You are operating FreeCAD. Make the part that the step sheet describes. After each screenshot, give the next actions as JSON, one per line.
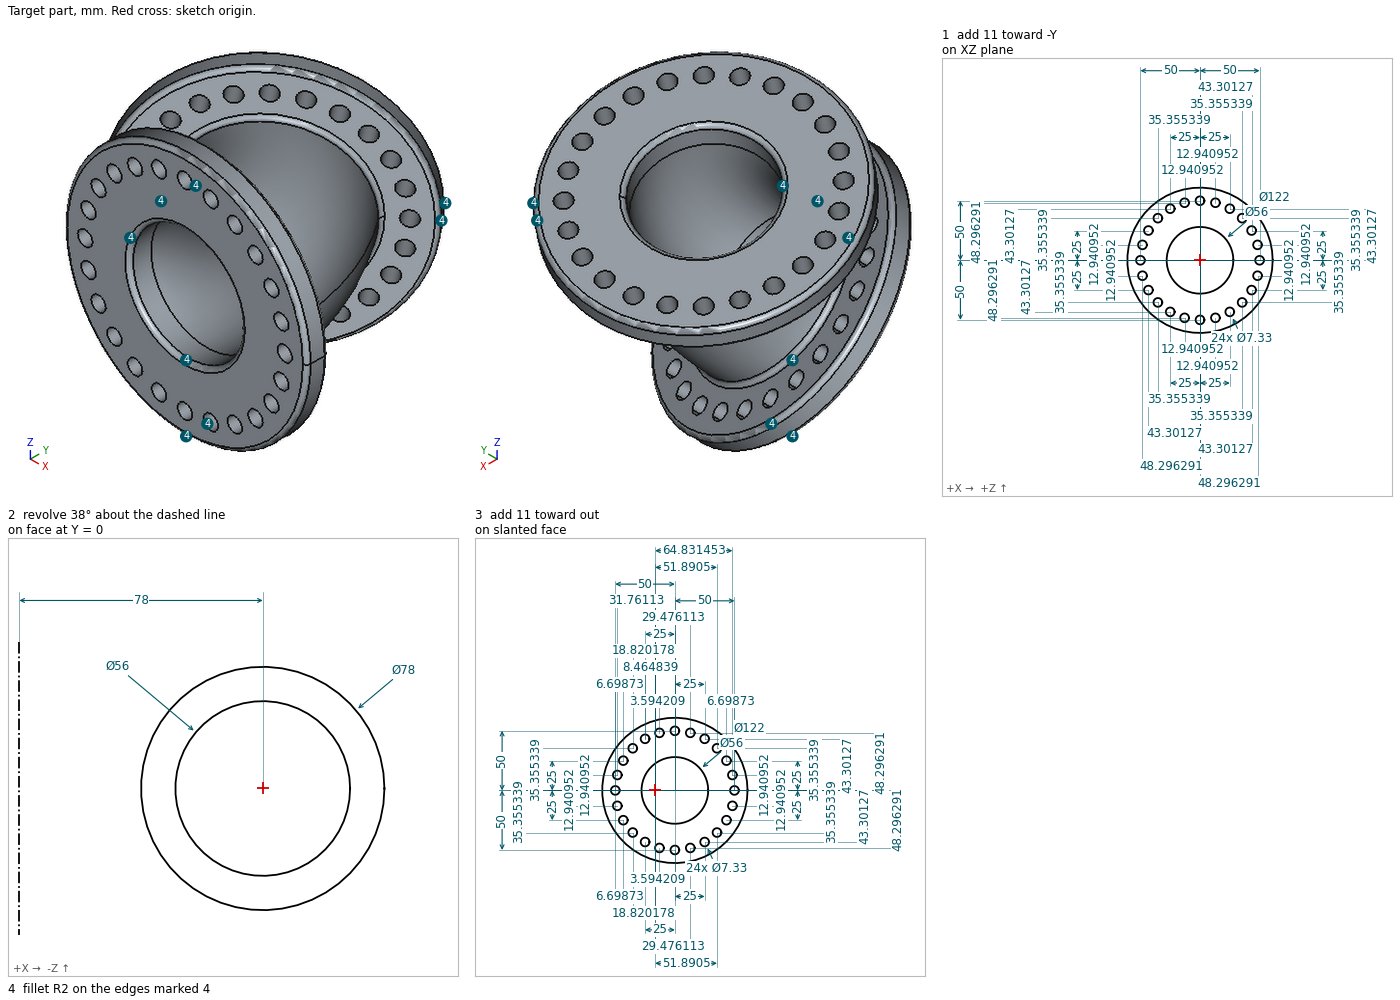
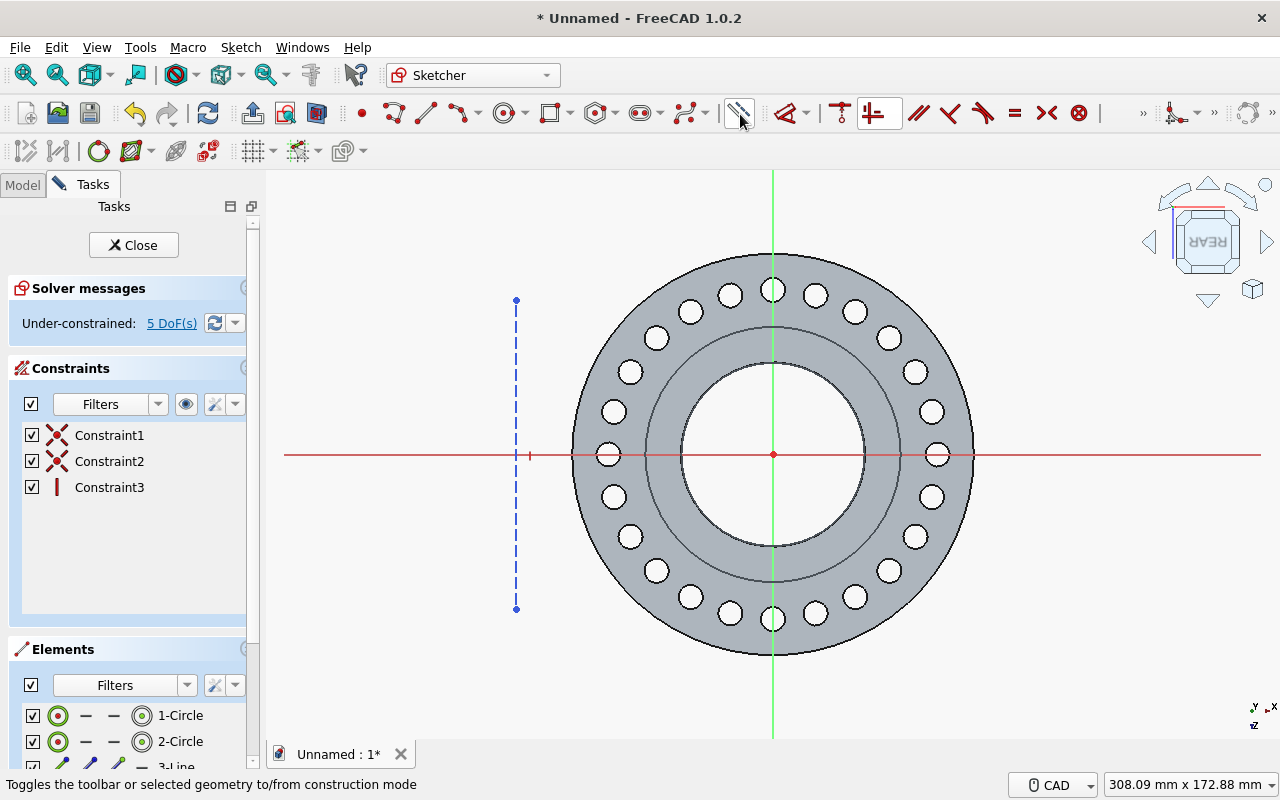
{"action": "left_click", "coordinate": [786, 114]}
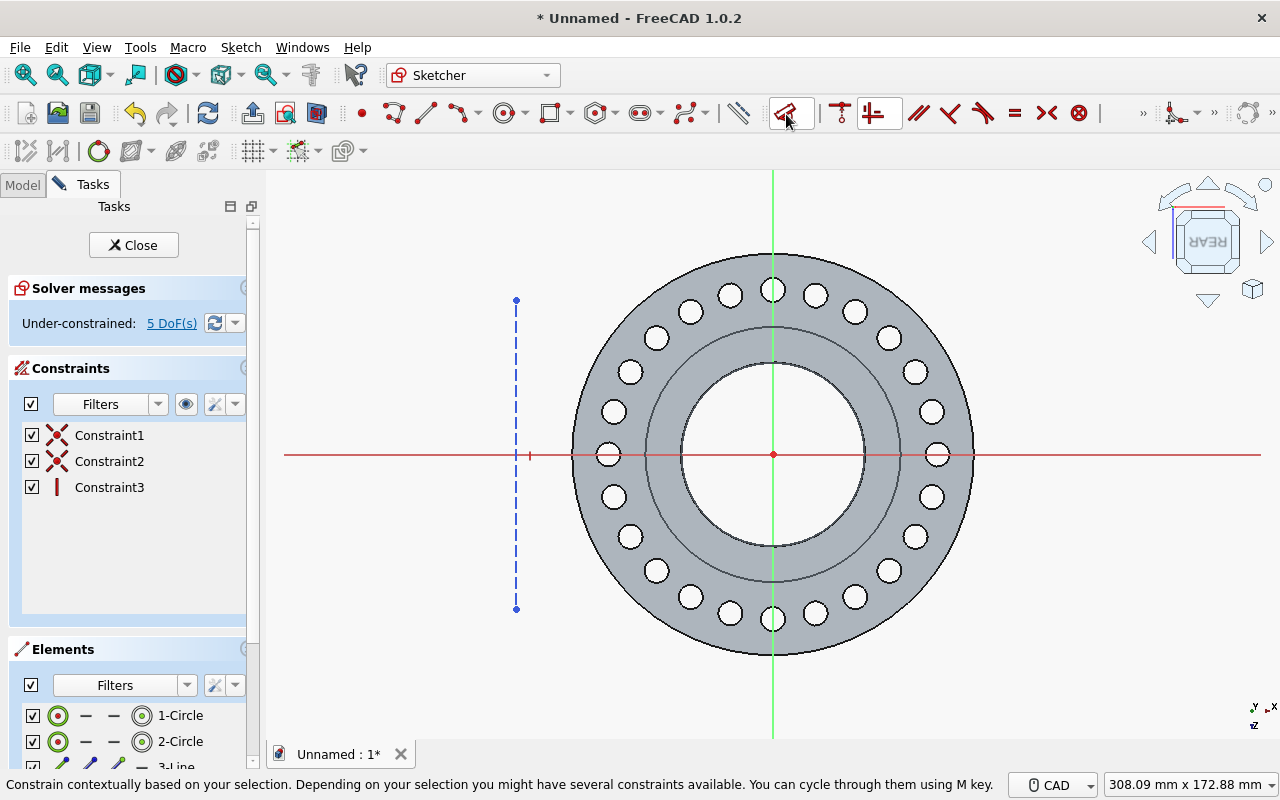
{"action": "left_click", "coordinate": [863, 364]}
{"action": "left_click", "coordinate": [886, 341]}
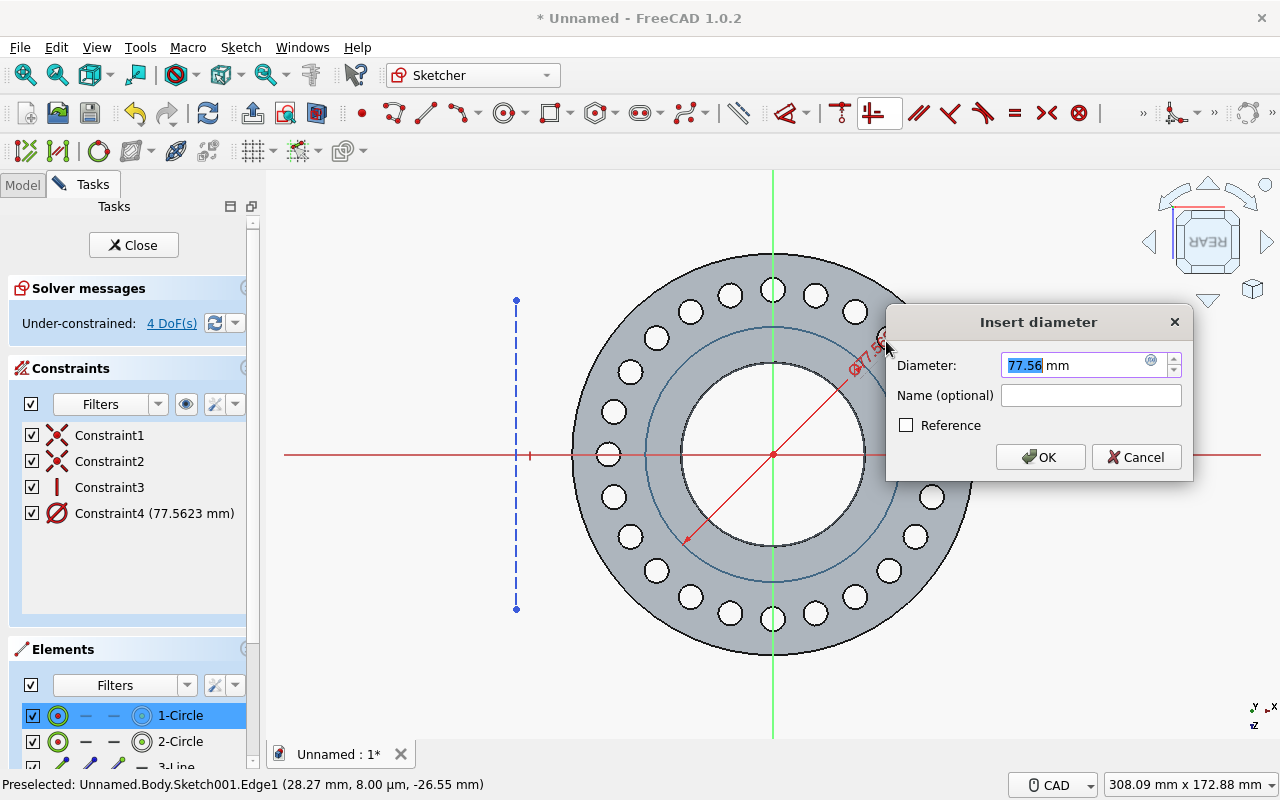
{"action": "type", "text": "78"}
{"action": "key", "text": "Return"}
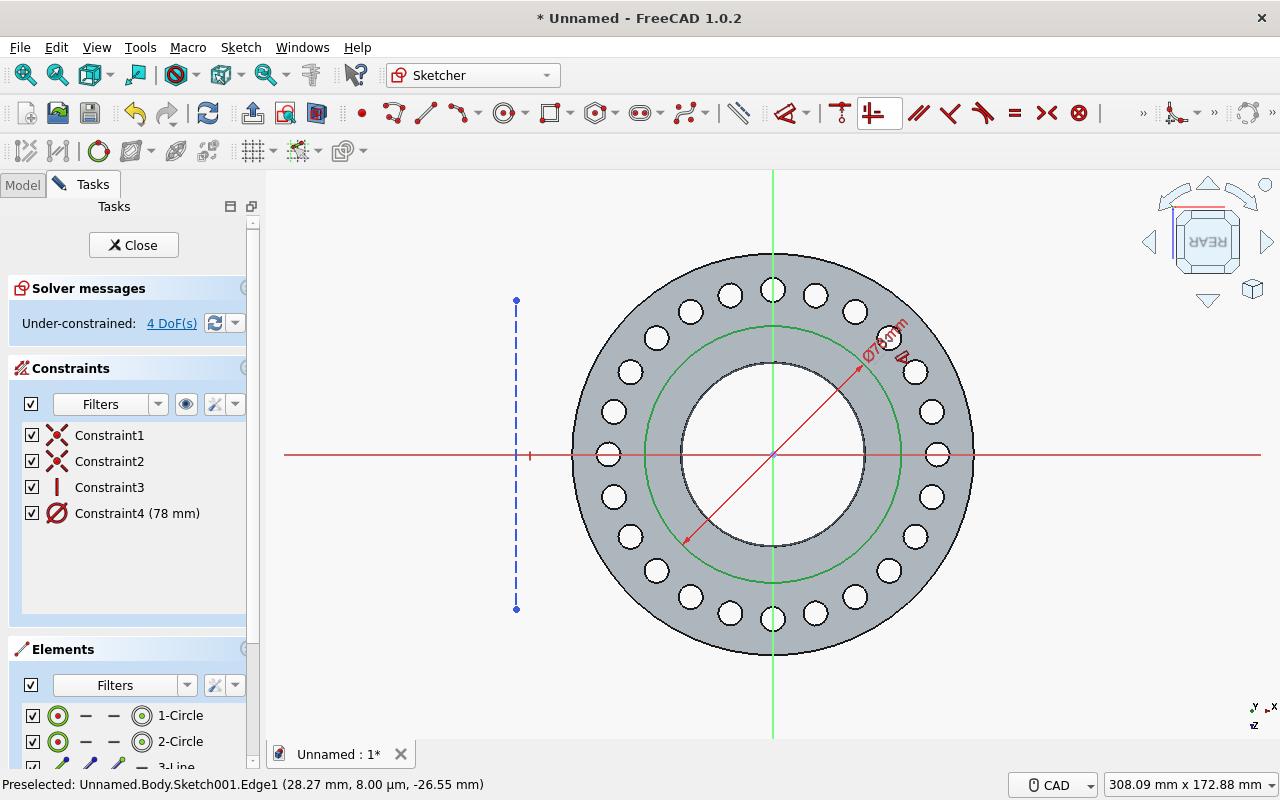
{"action": "left_click", "coordinate": [838, 390]}
{"action": "left_click", "coordinate": [914, 414]}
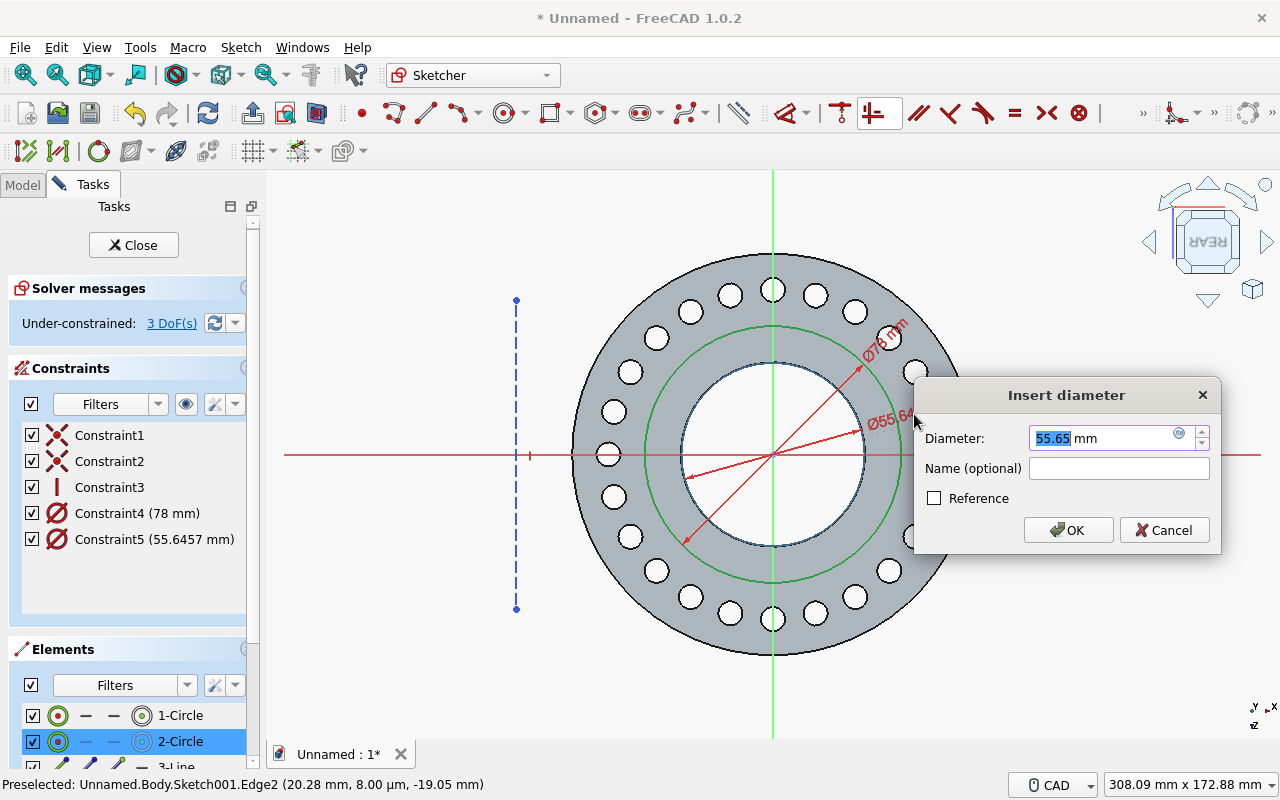
{"action": "type", "text": "56"}
{"action": "key", "text": "Return"}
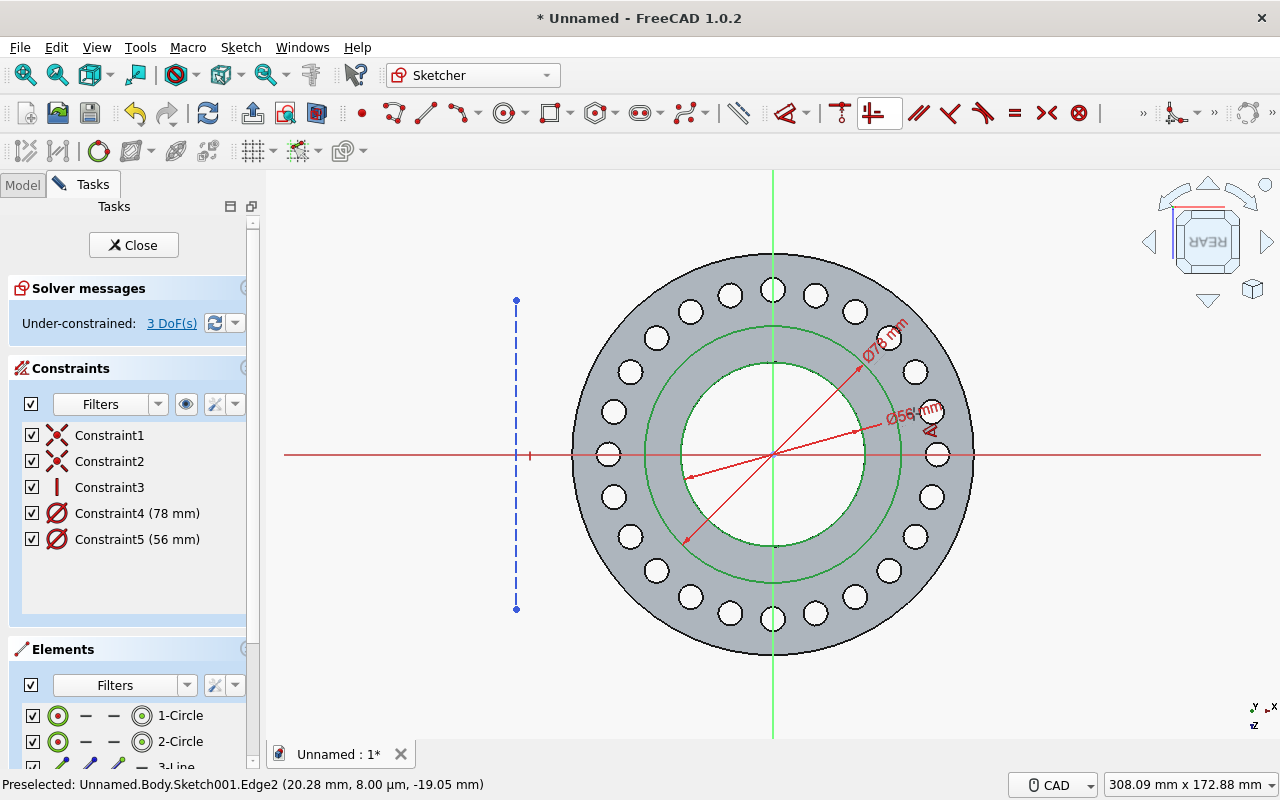
{"action": "left_click", "coordinate": [516, 301]}
{"action": "left_click", "coordinate": [644, 267]}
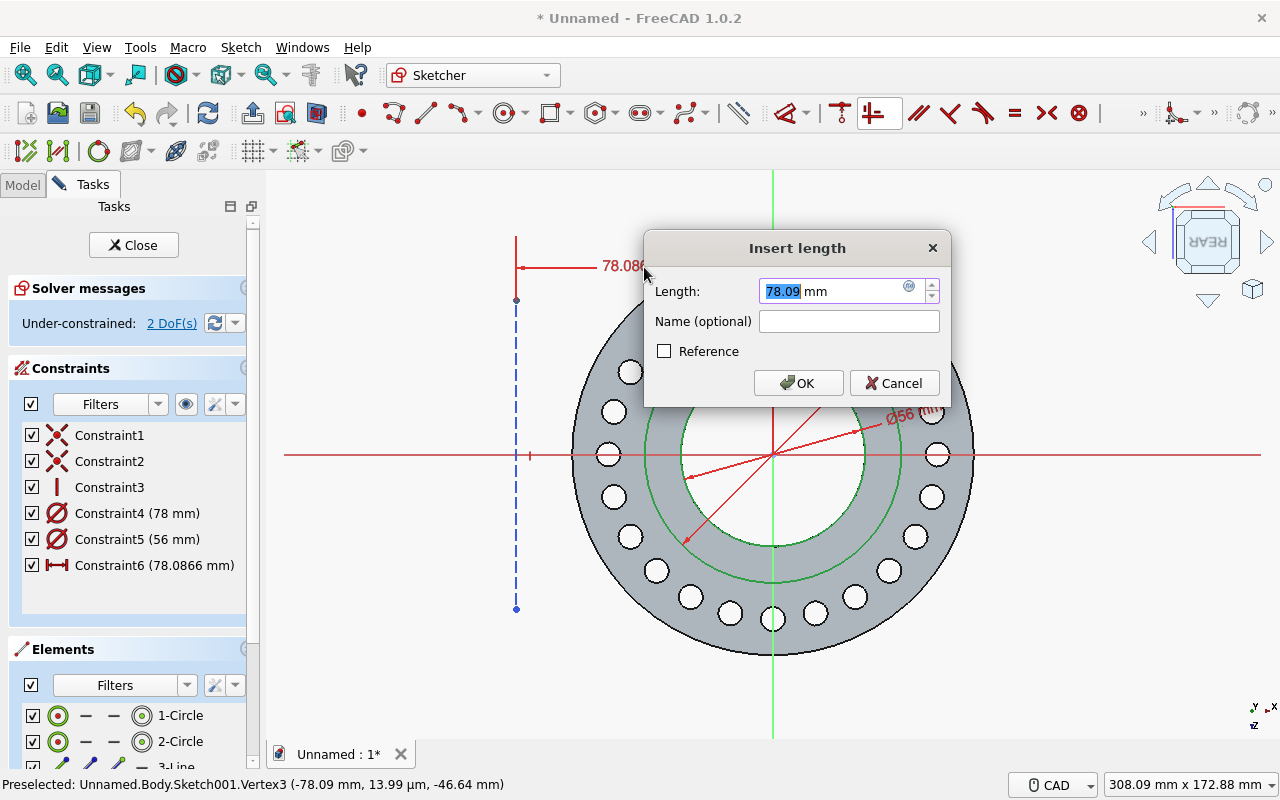
{"action": "type", "text": "78"}
{"action": "key", "text": "Return"}
{"action": "key", "text": "Escape"}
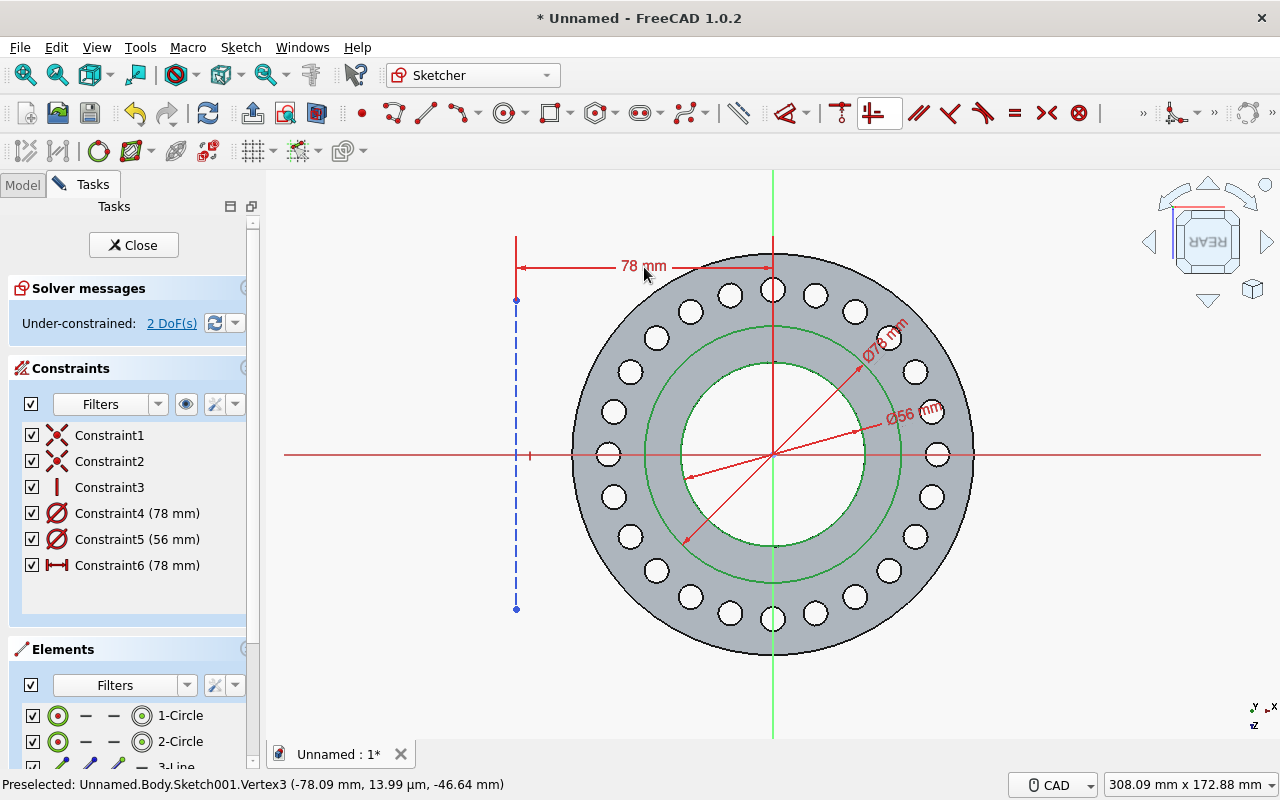
{"action": "left_click", "coordinate": [134, 245]}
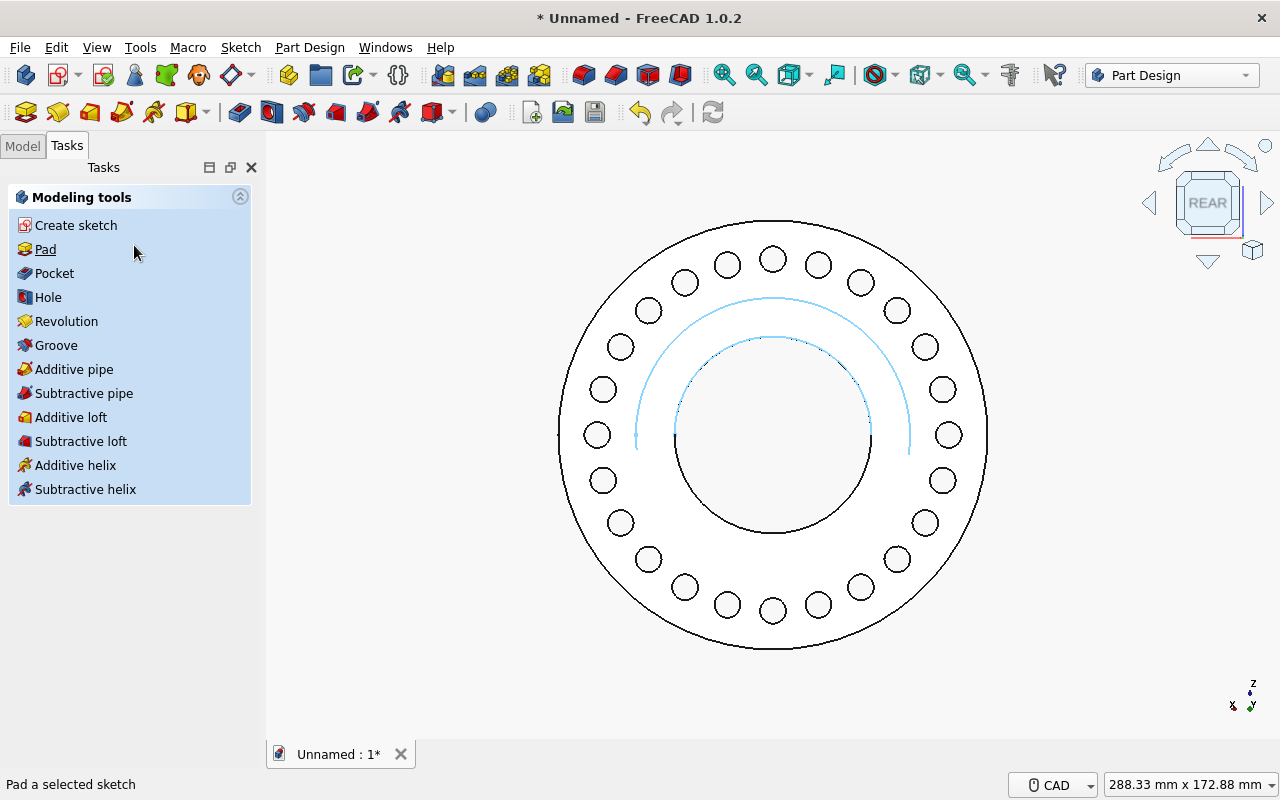
{"action": "left_click", "coordinate": [58, 112]}